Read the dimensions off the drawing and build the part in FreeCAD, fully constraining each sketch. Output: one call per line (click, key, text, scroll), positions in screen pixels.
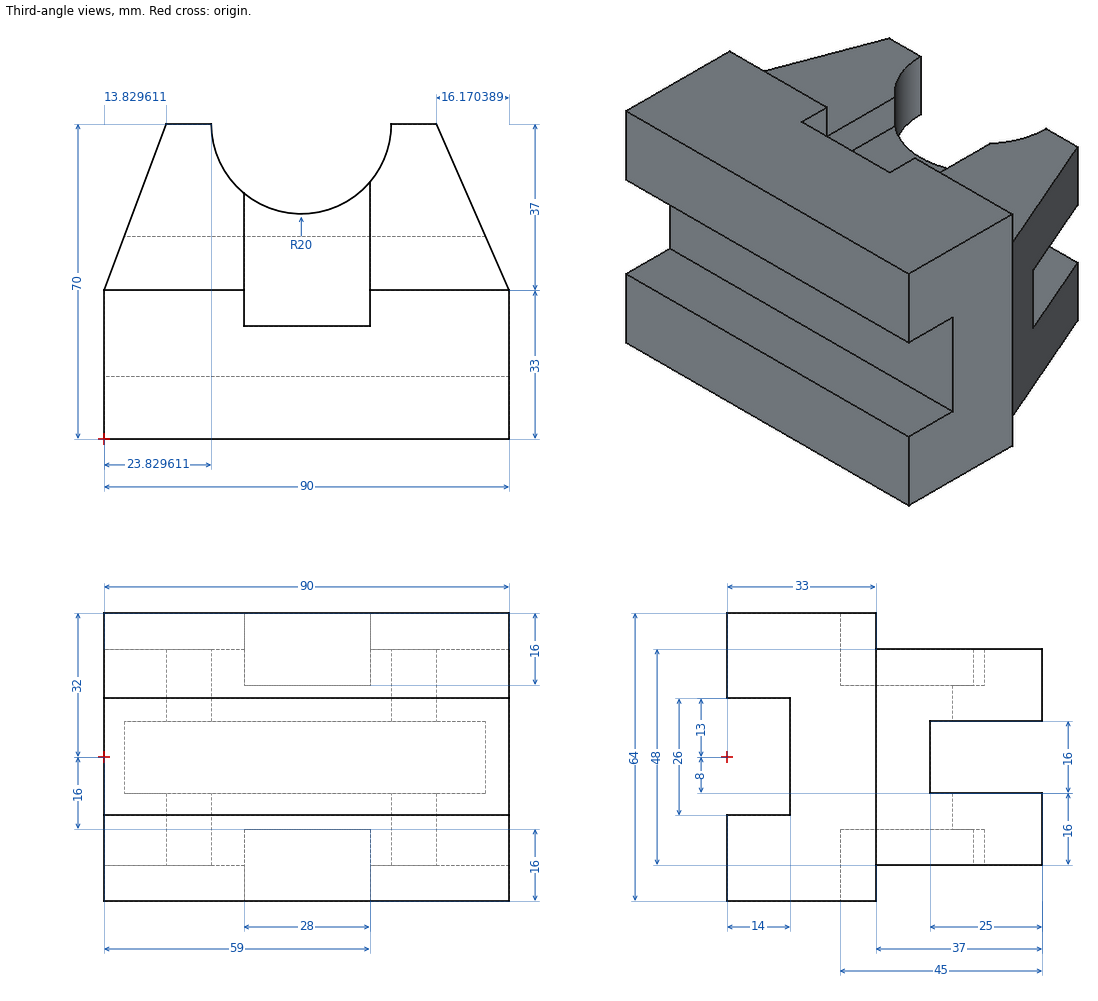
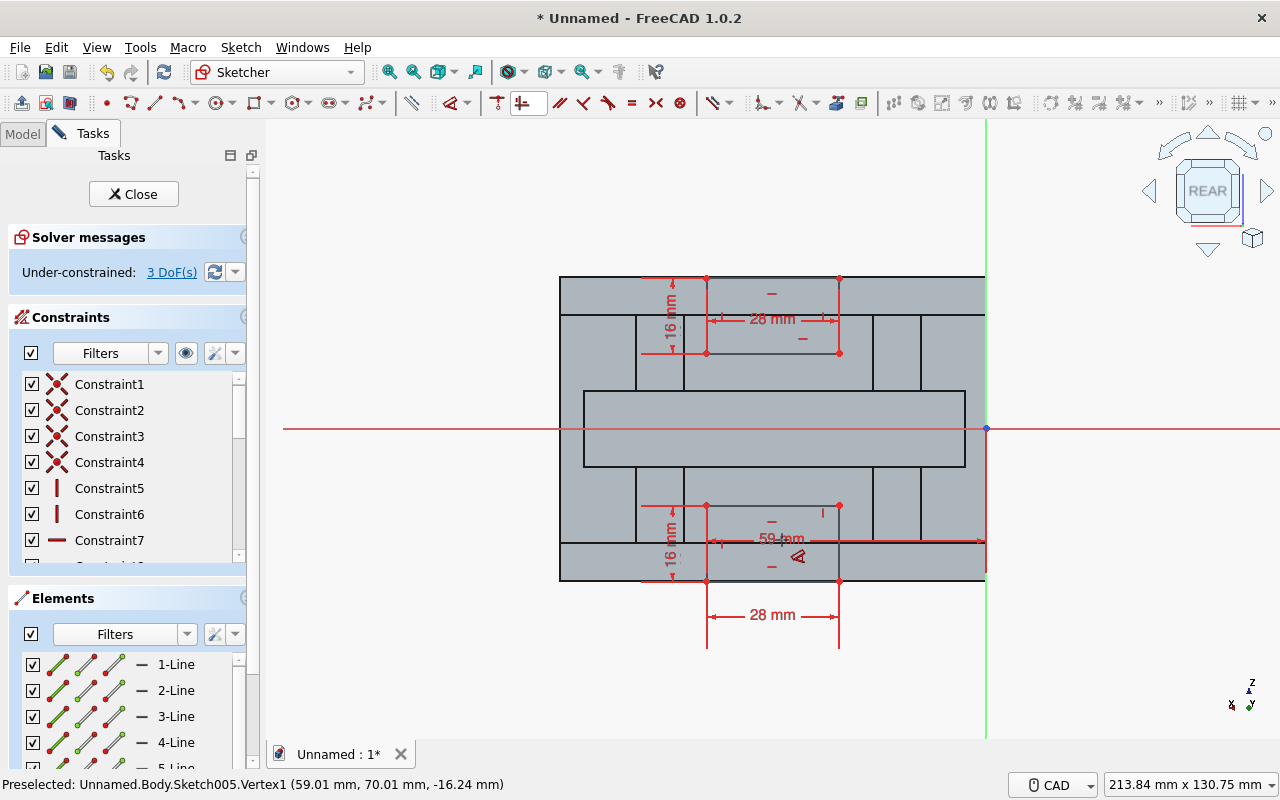
click(707, 506)
click(1020, 467)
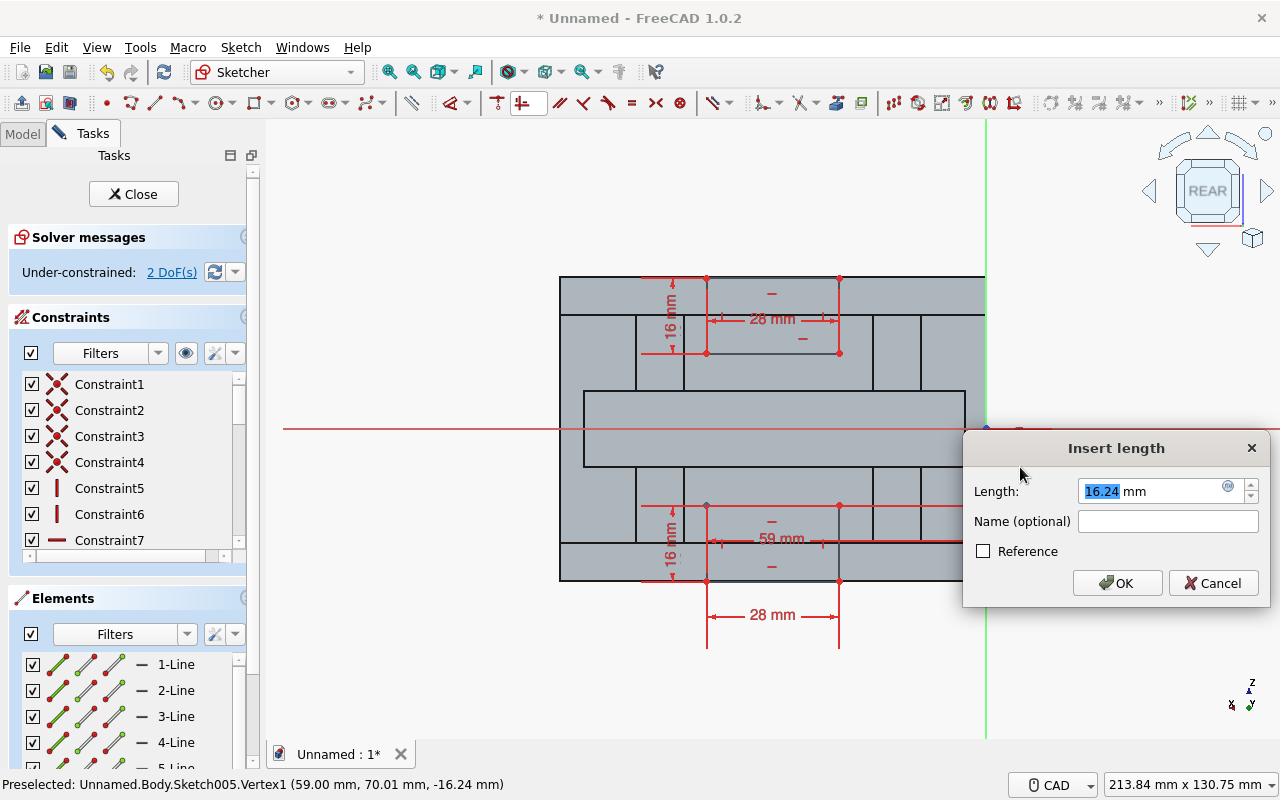
text(16)
key(Return)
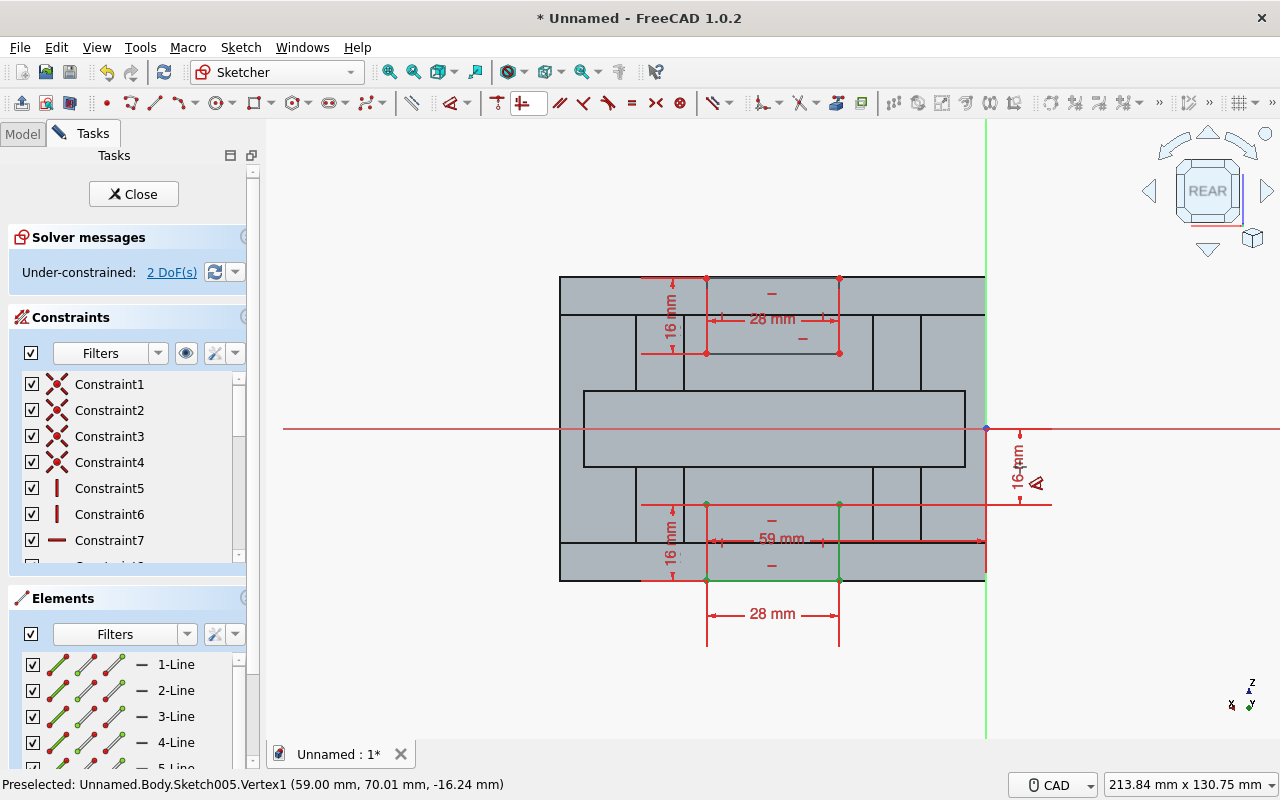
click(707, 278)
click(846, 244)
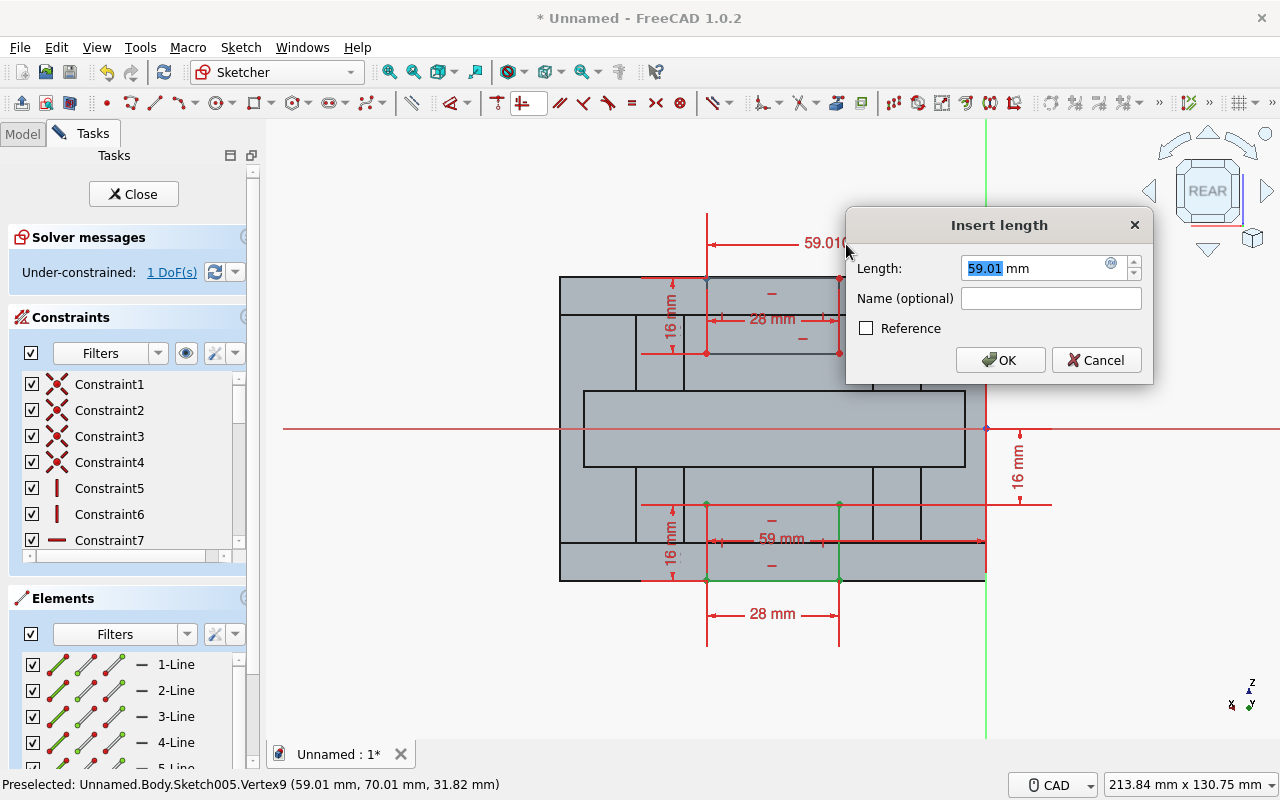
text(59)
key(Return)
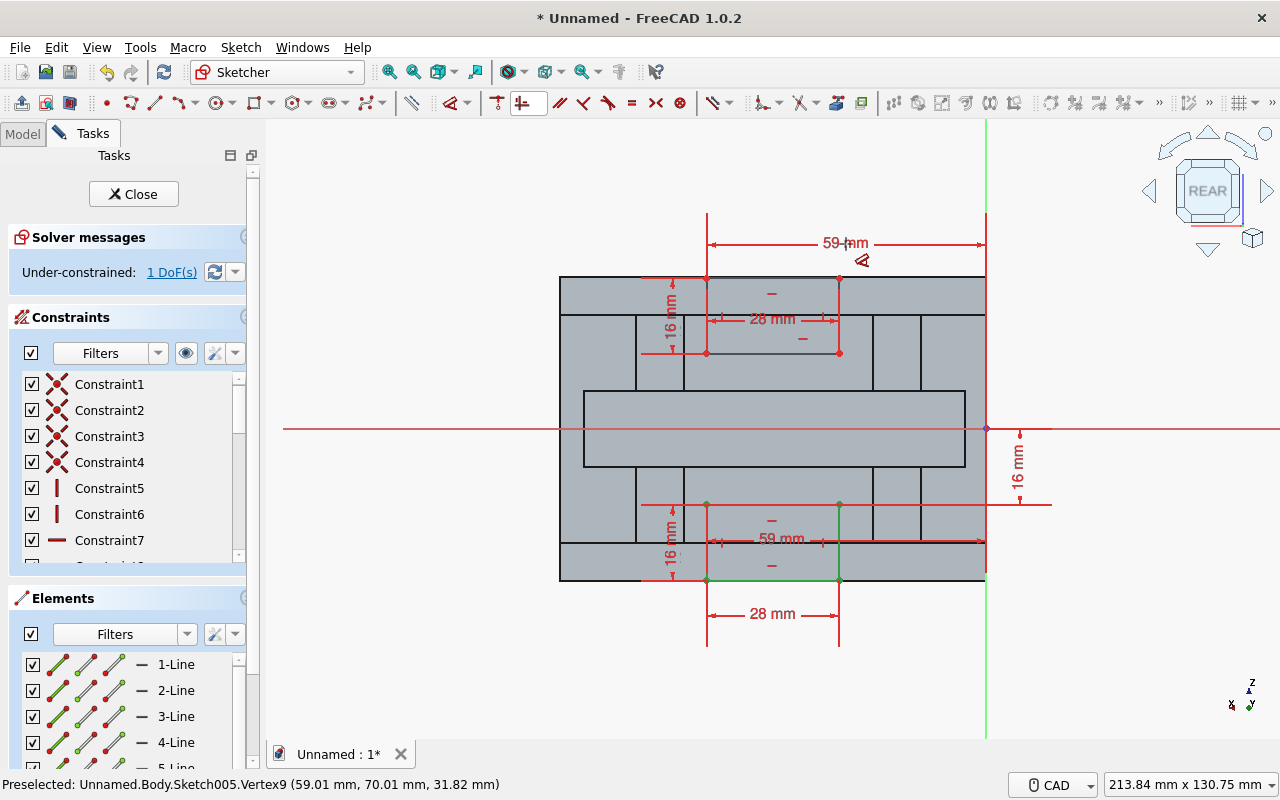
click(707, 278)
click(1020, 354)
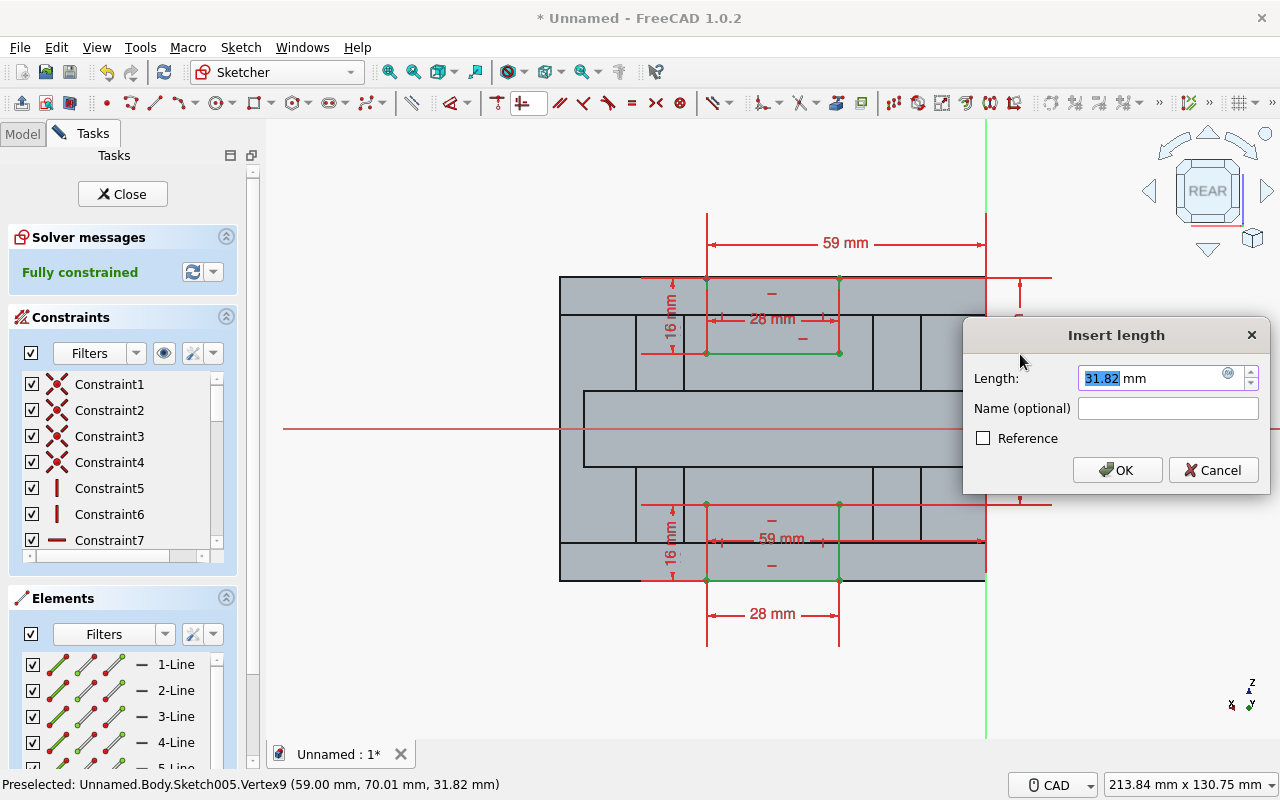
text(32)
key(Return)
key(Escape)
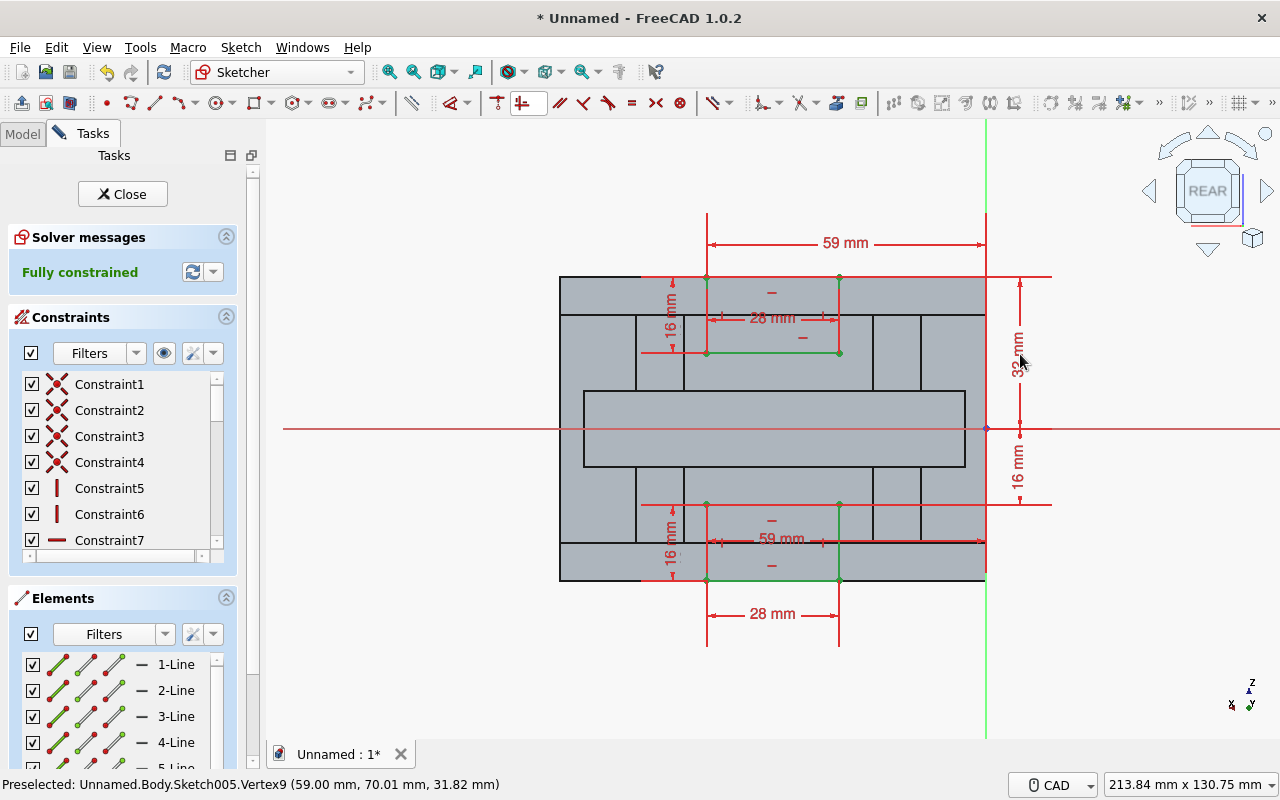
click(123, 194)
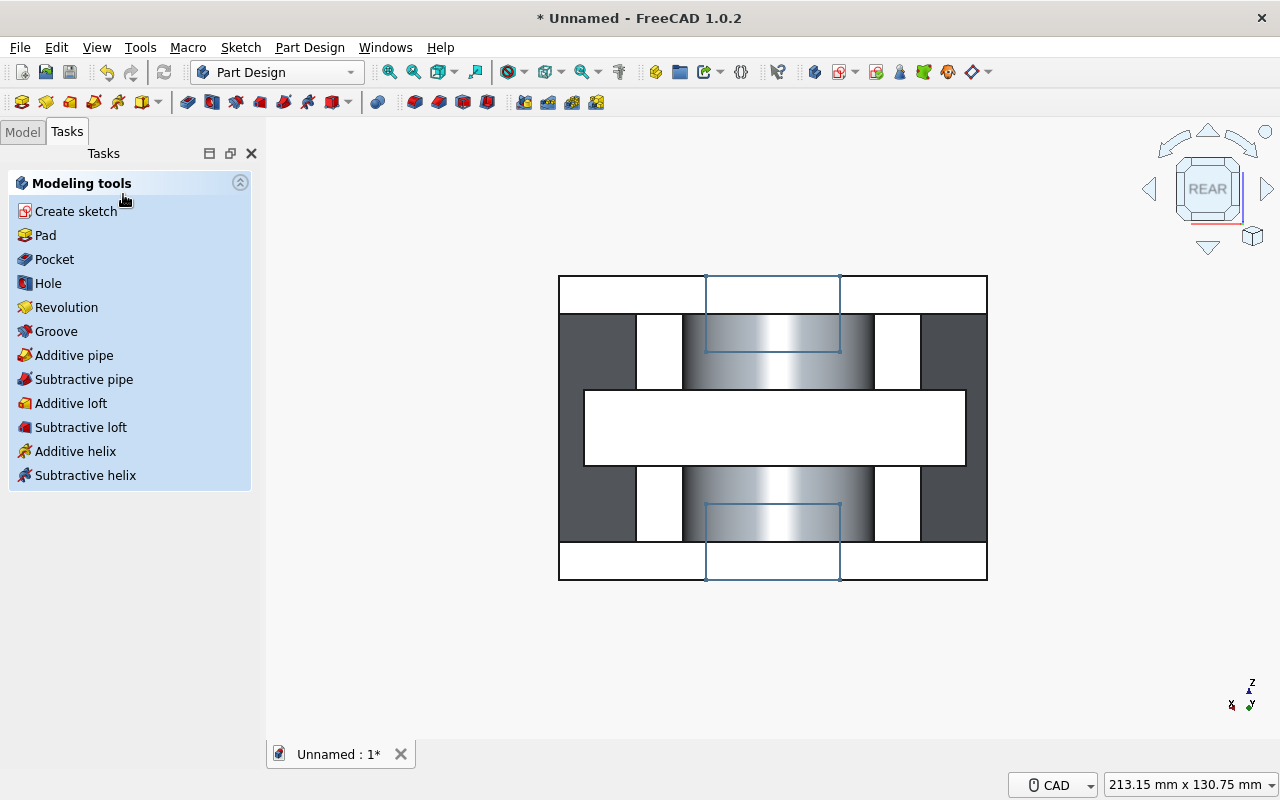
click(188, 102)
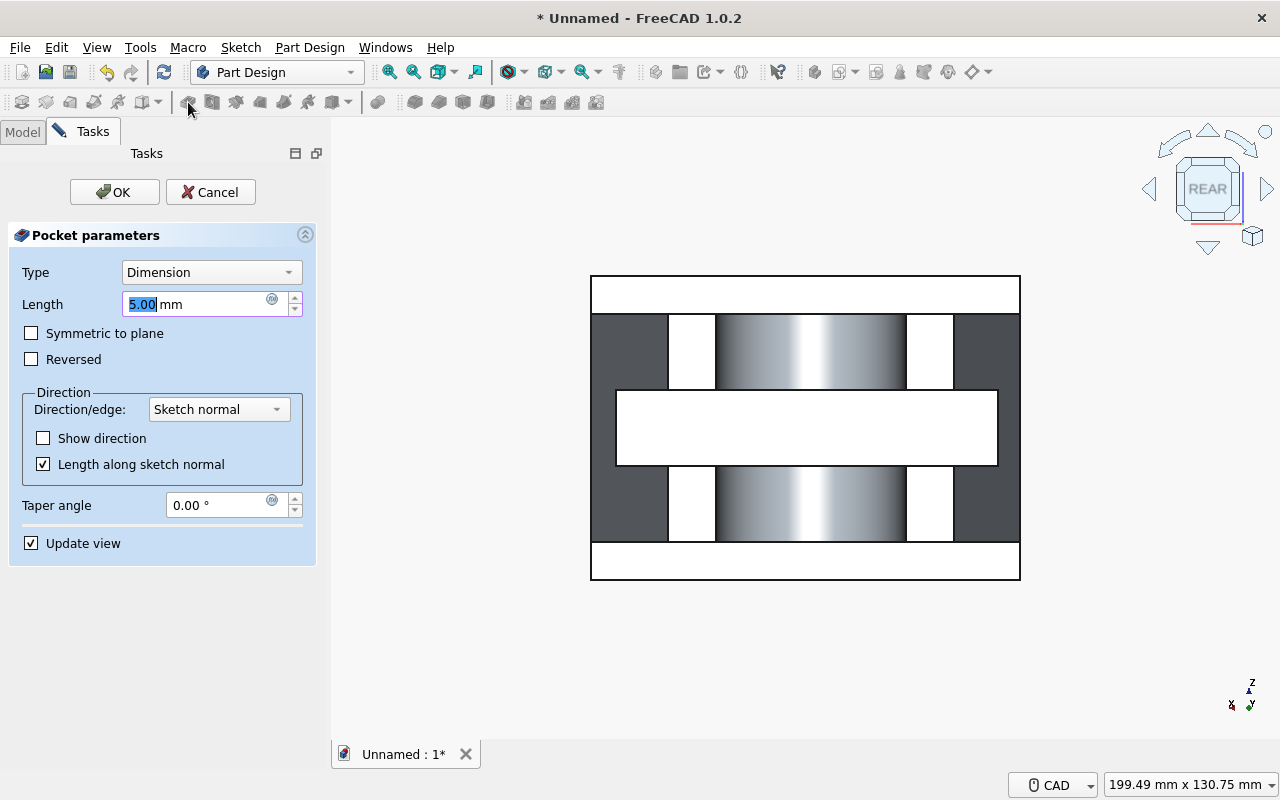
text(45)
key(Tab)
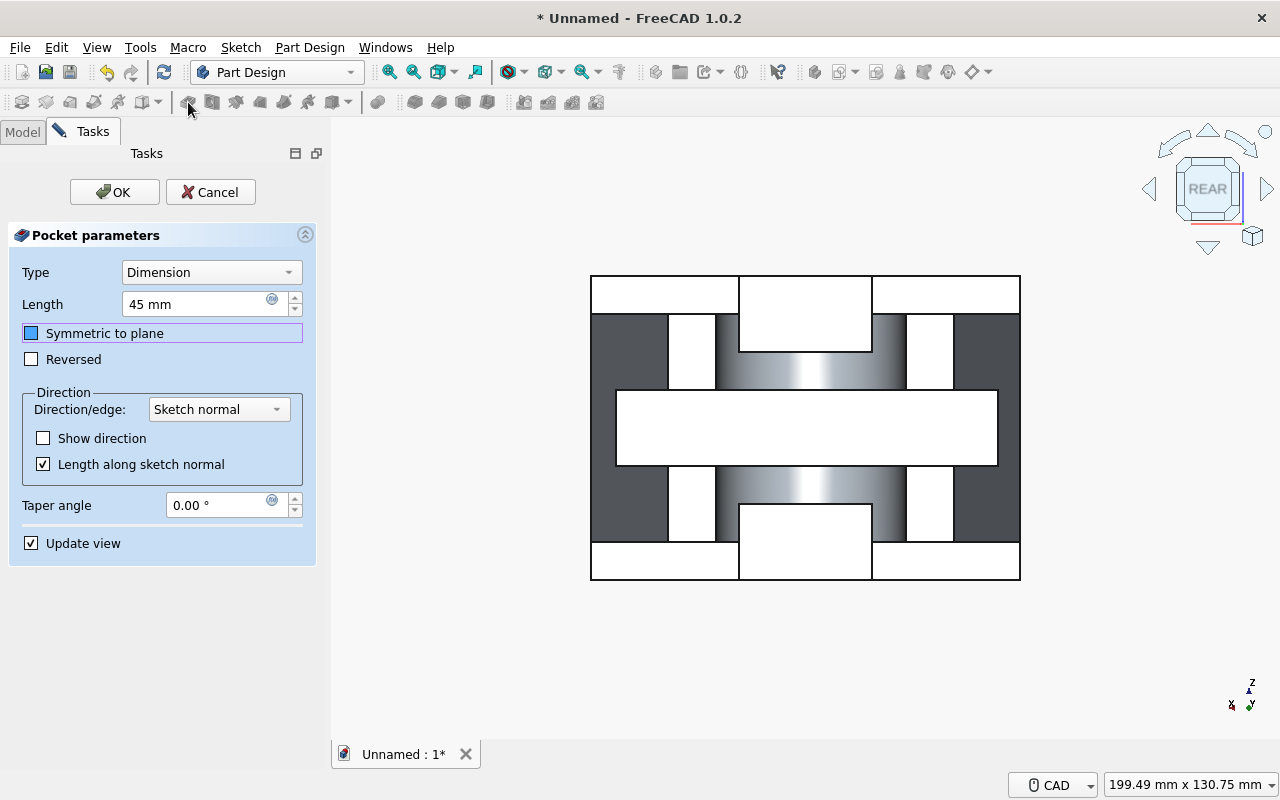
click(115, 192)